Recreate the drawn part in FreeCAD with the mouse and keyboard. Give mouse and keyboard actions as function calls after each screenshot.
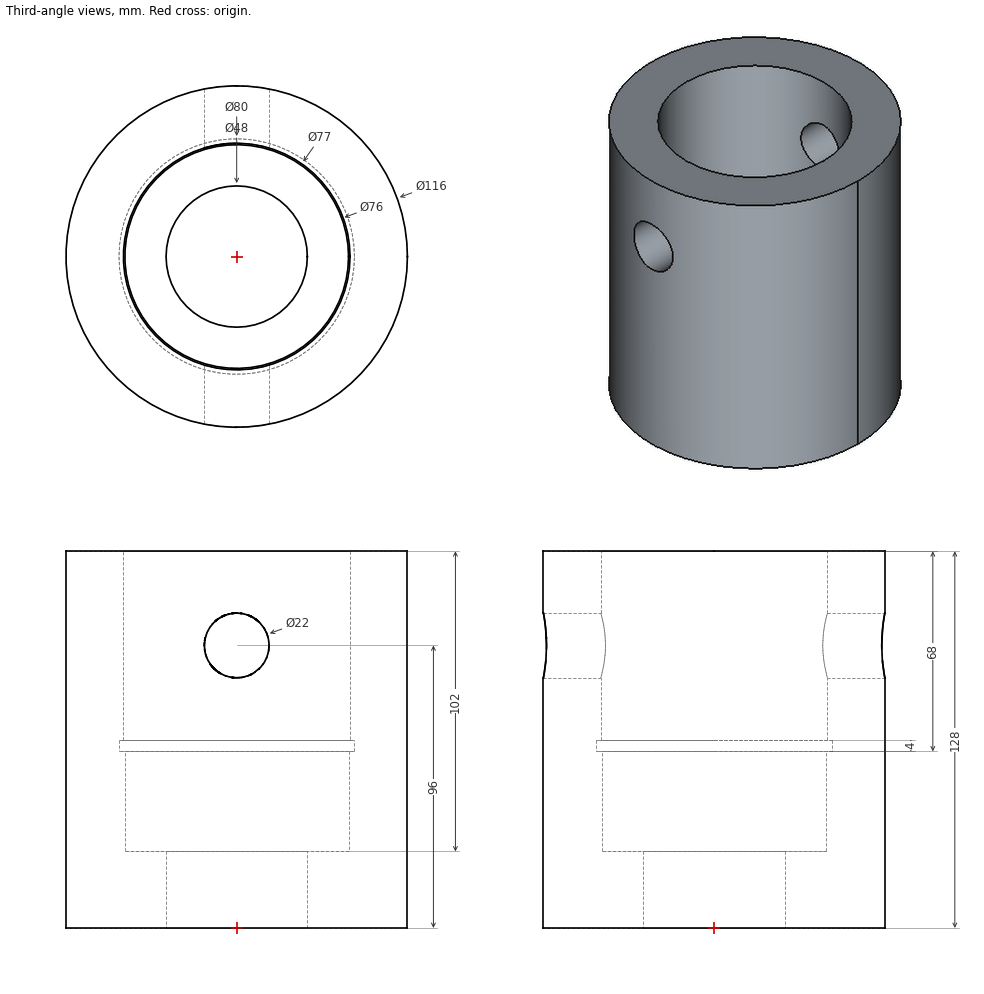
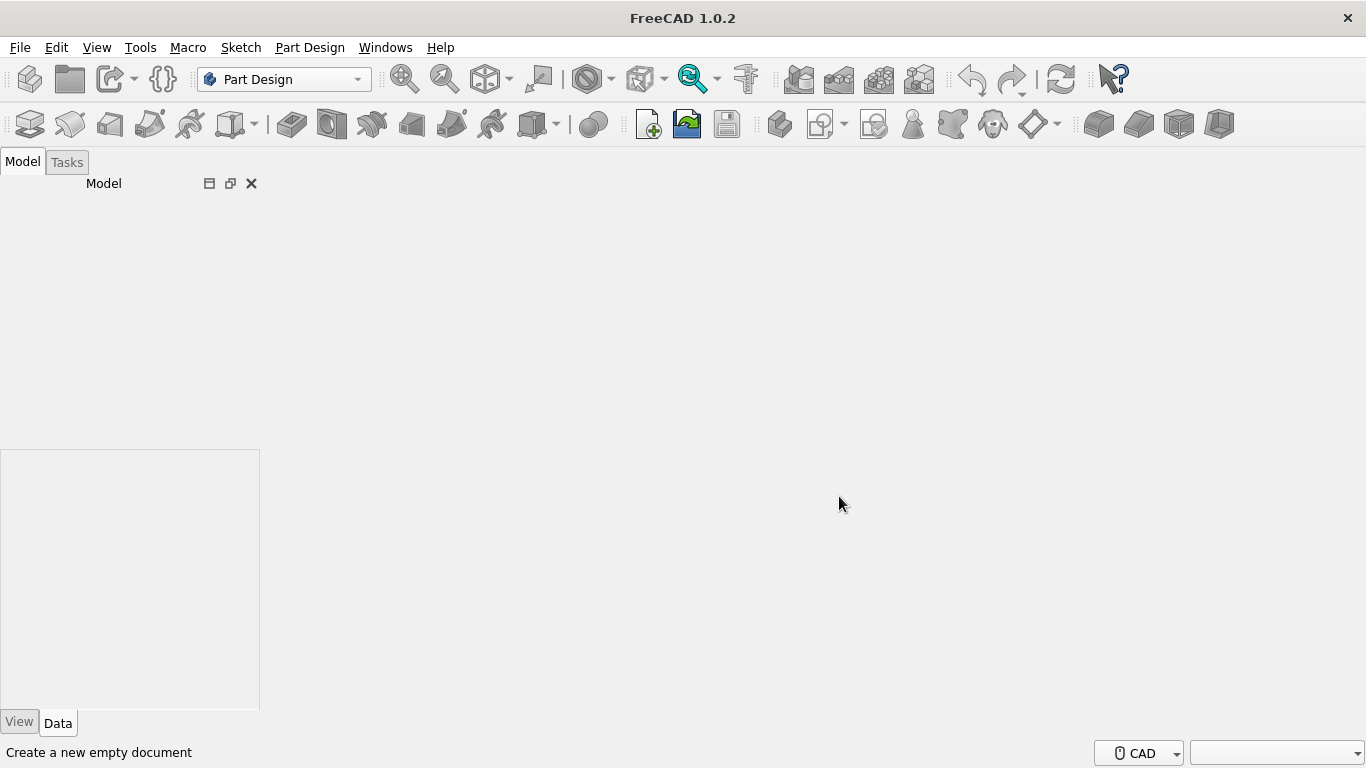
click(648, 124)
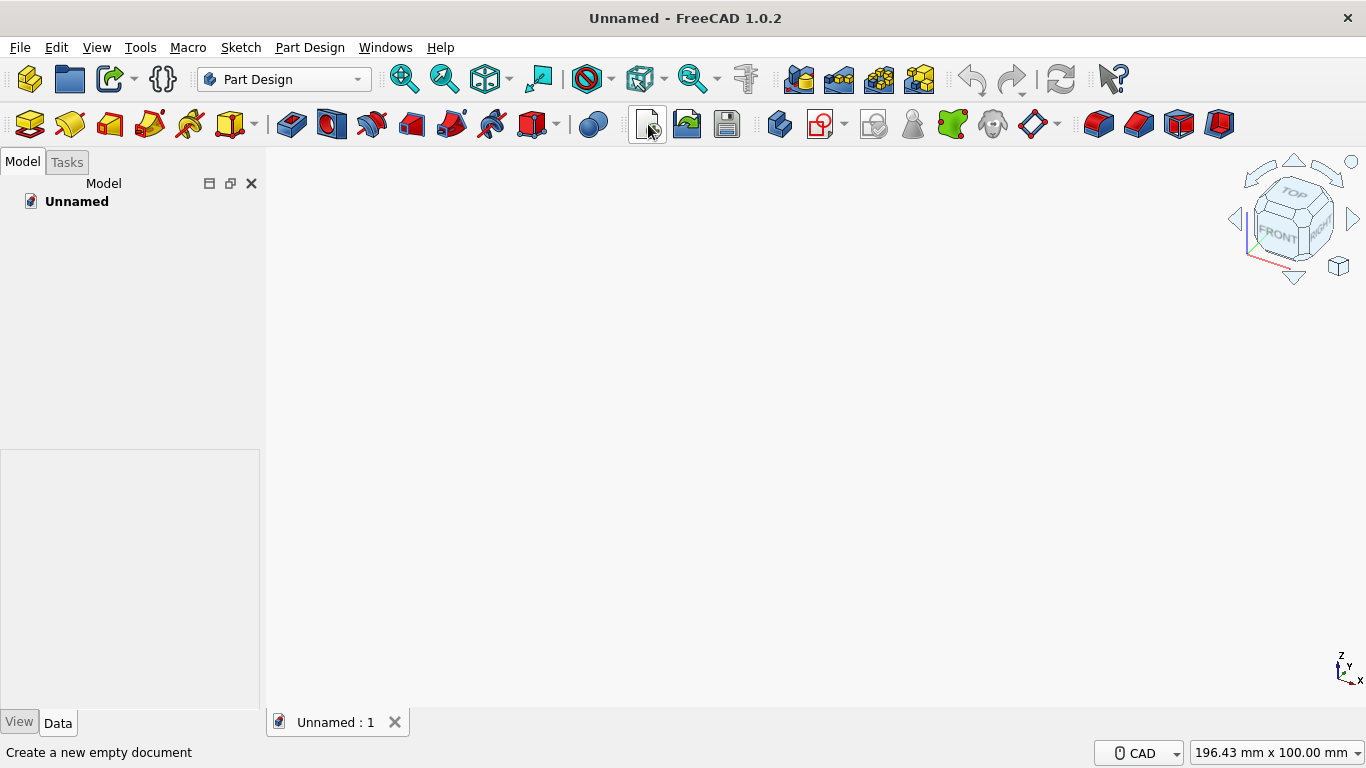
click(820, 124)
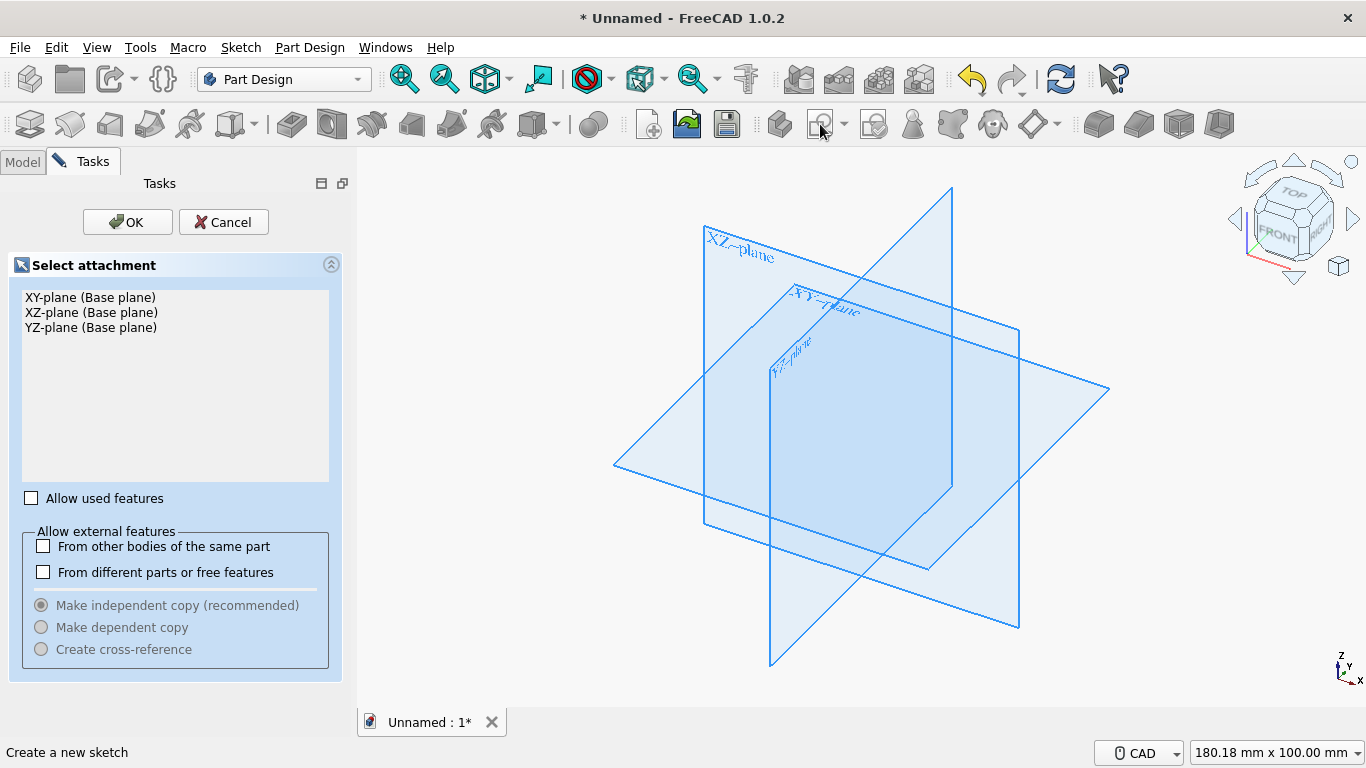
click(82, 298)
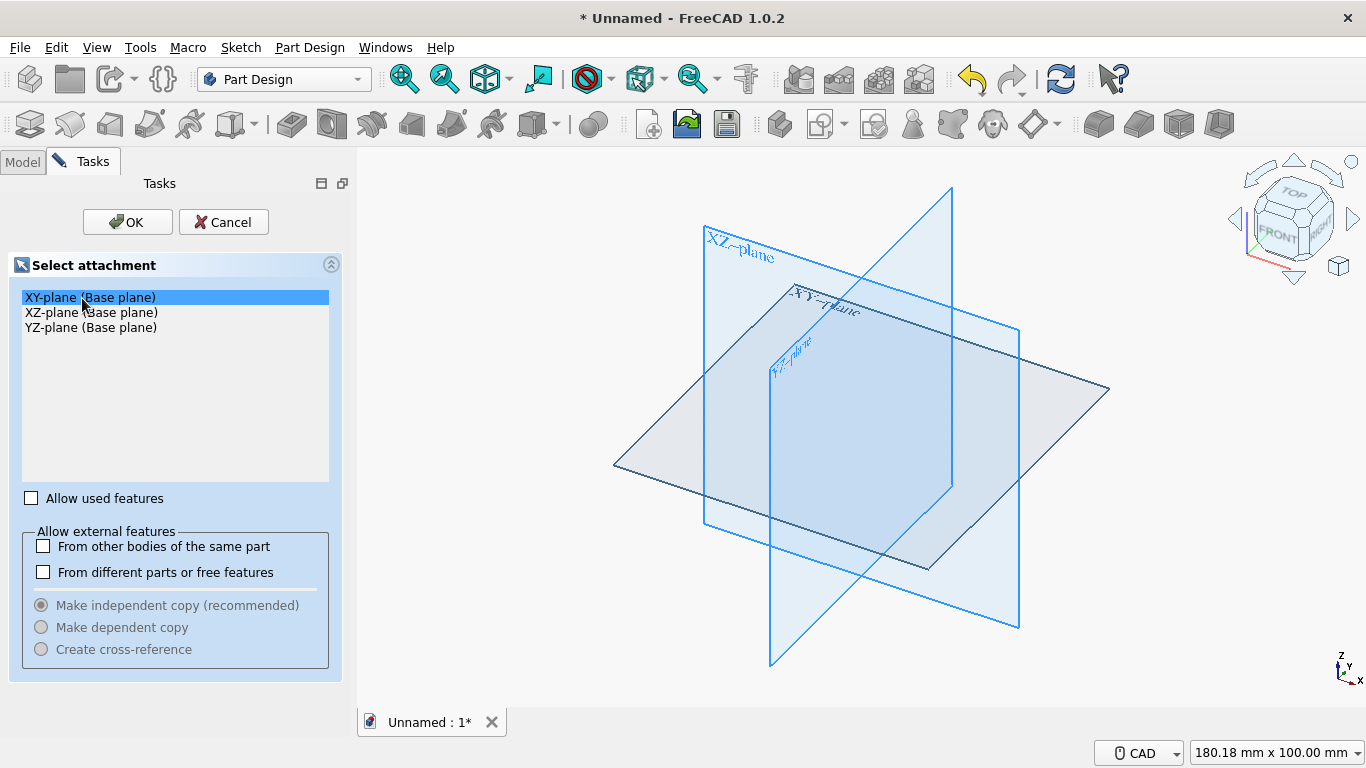
click(128, 222)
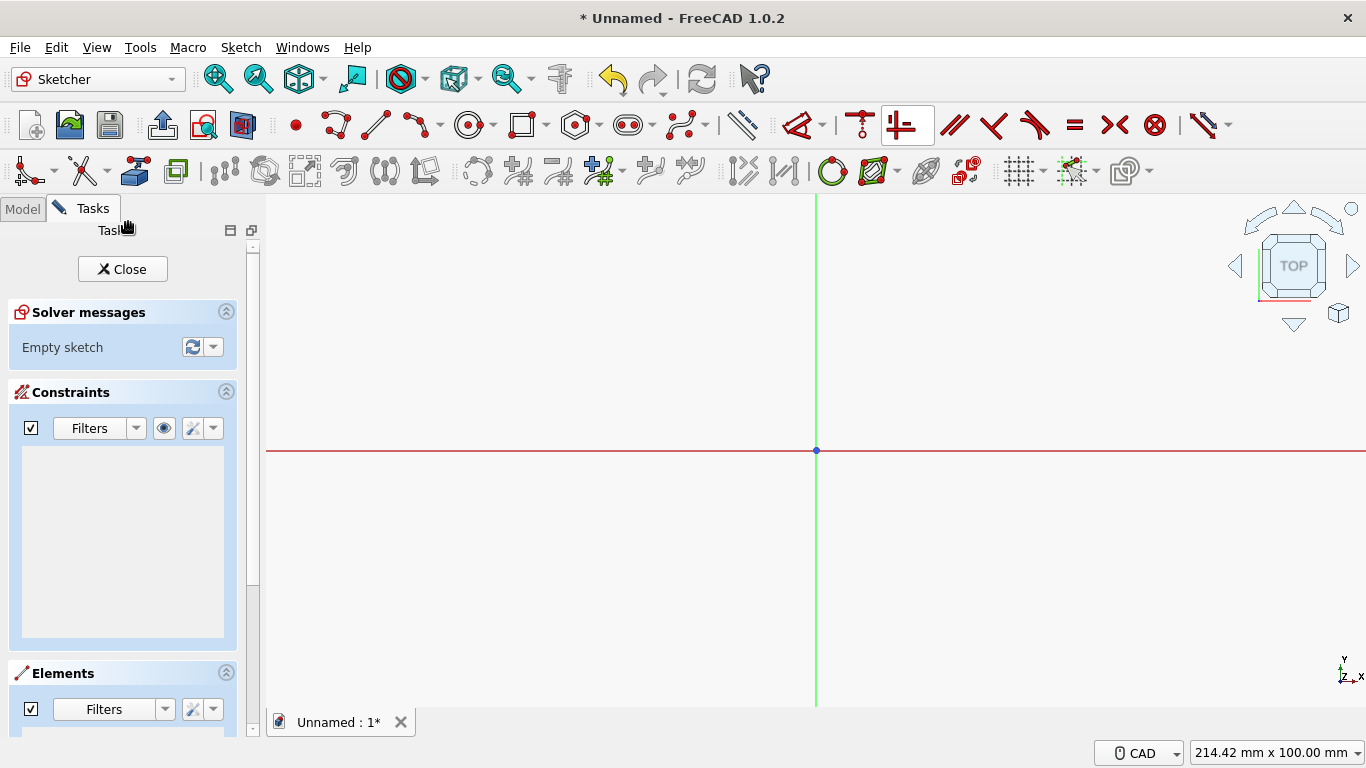
scroll(664, 451, down, 3)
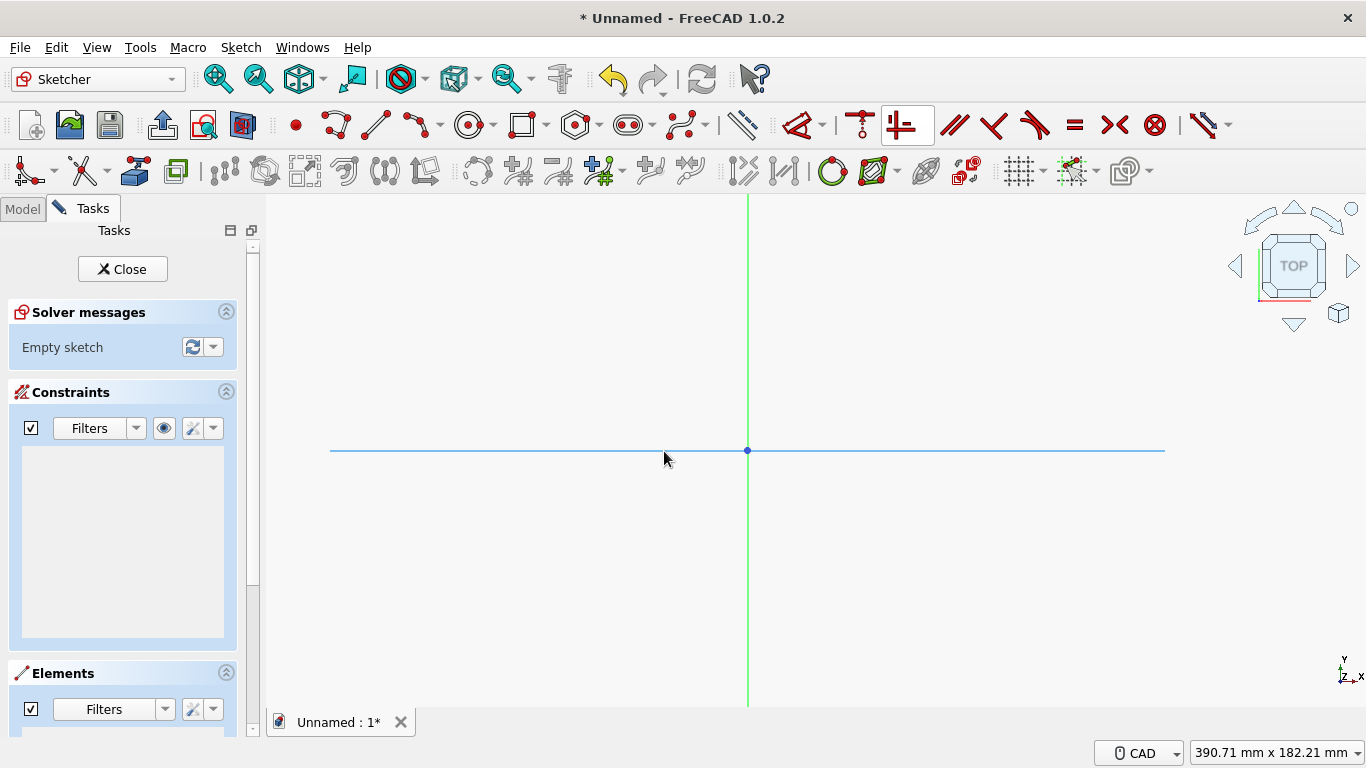
click(470, 126)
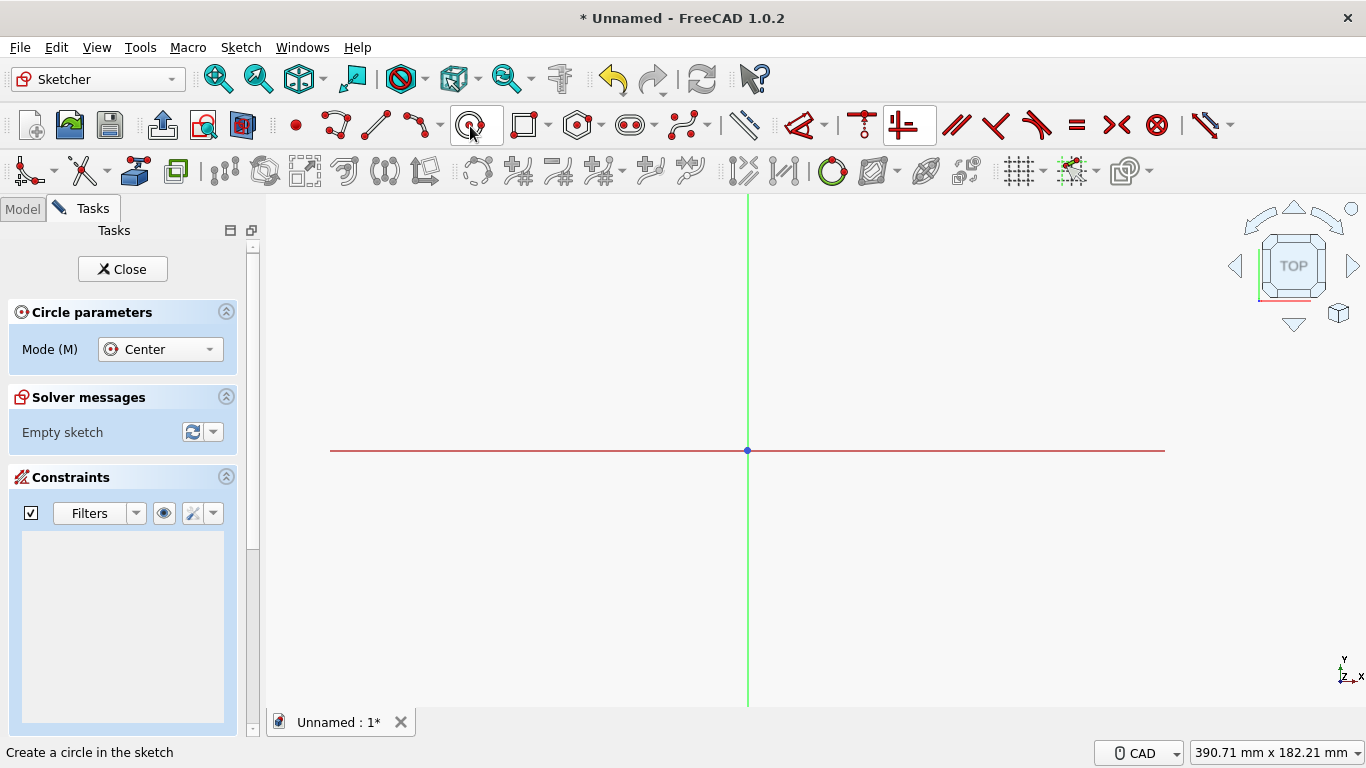
click(748, 451)
move(863, 335)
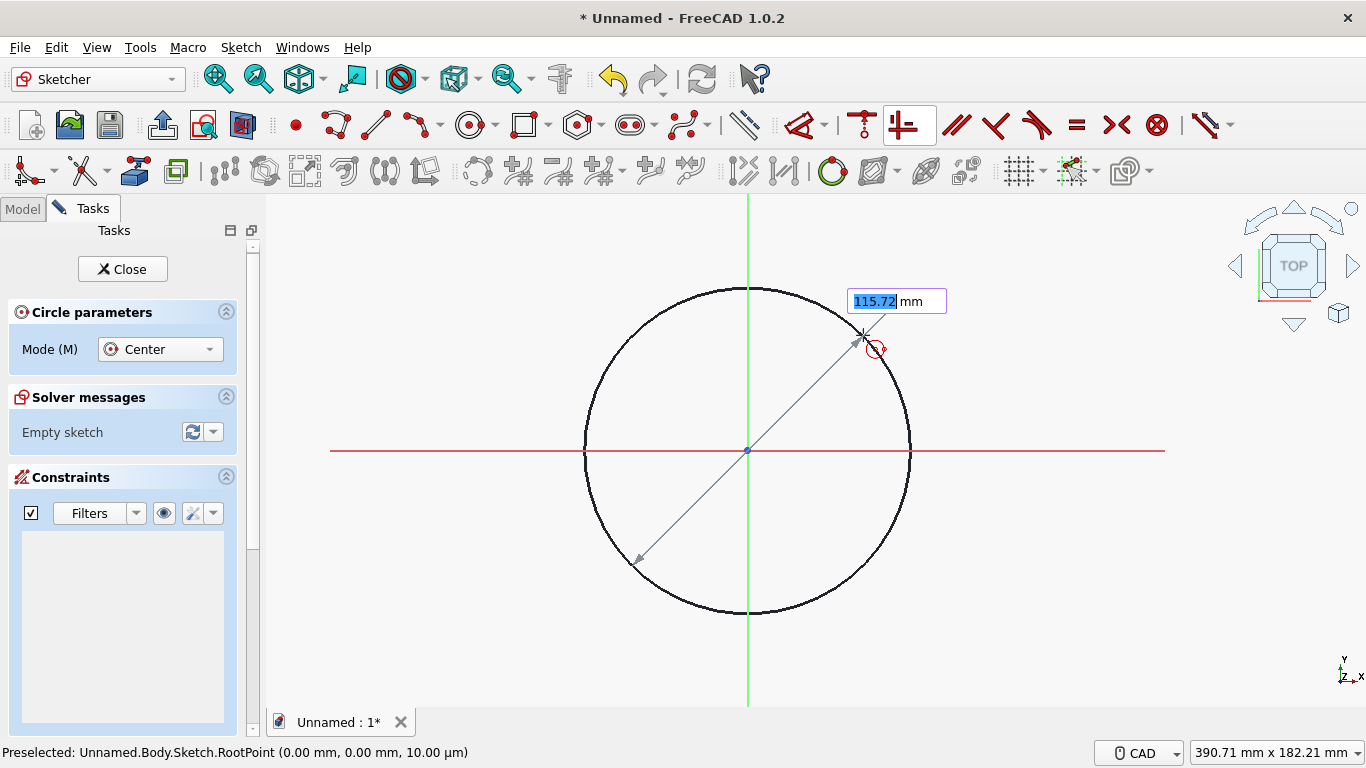
text(116)
key(Return)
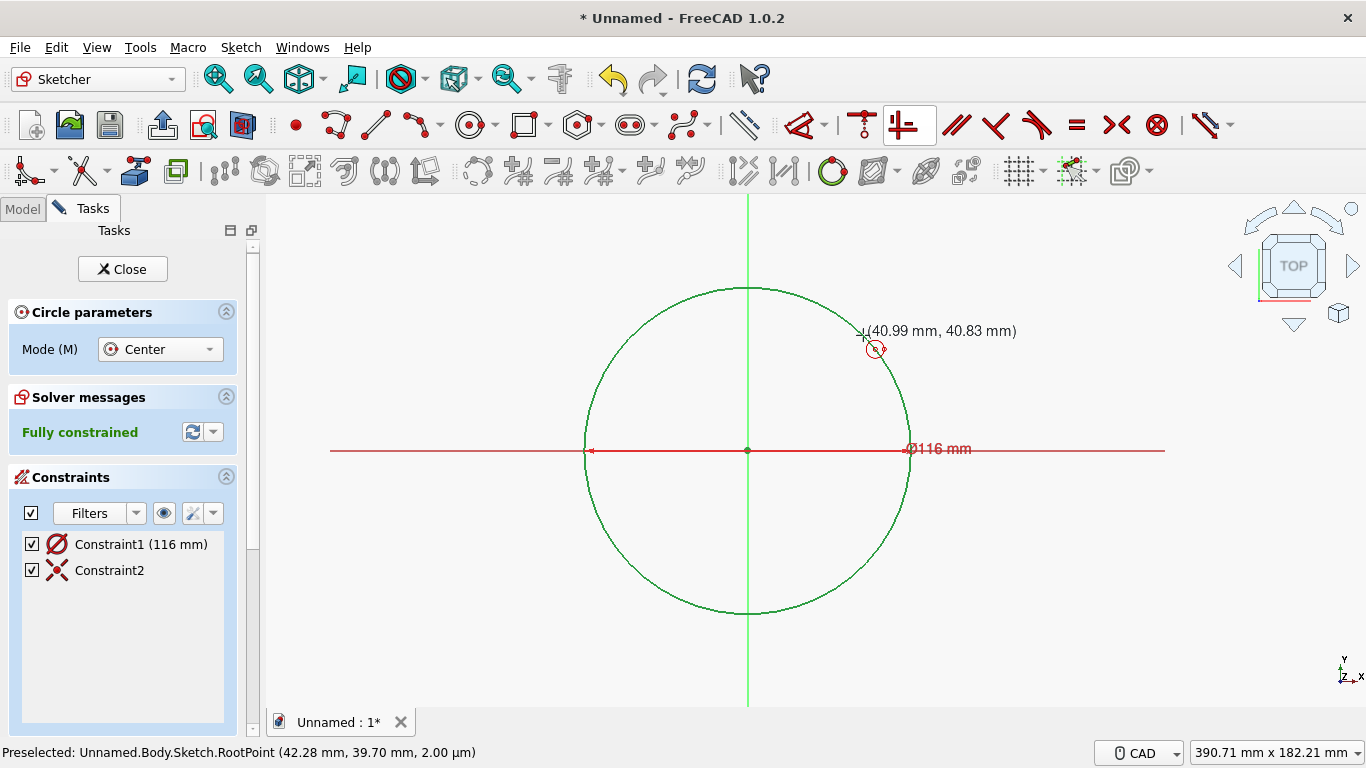
click(748, 451)
move(795, 403)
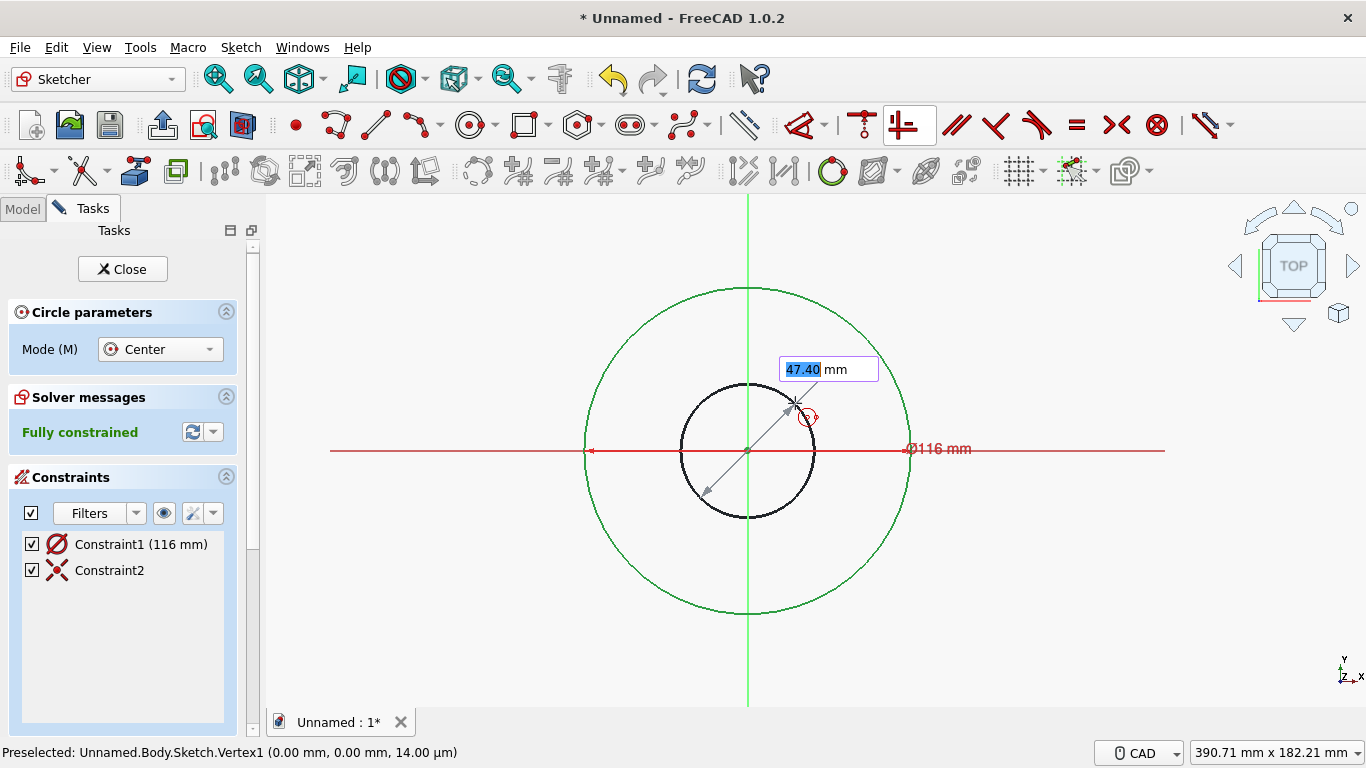
text(48)
key(Return)
key(Escape)